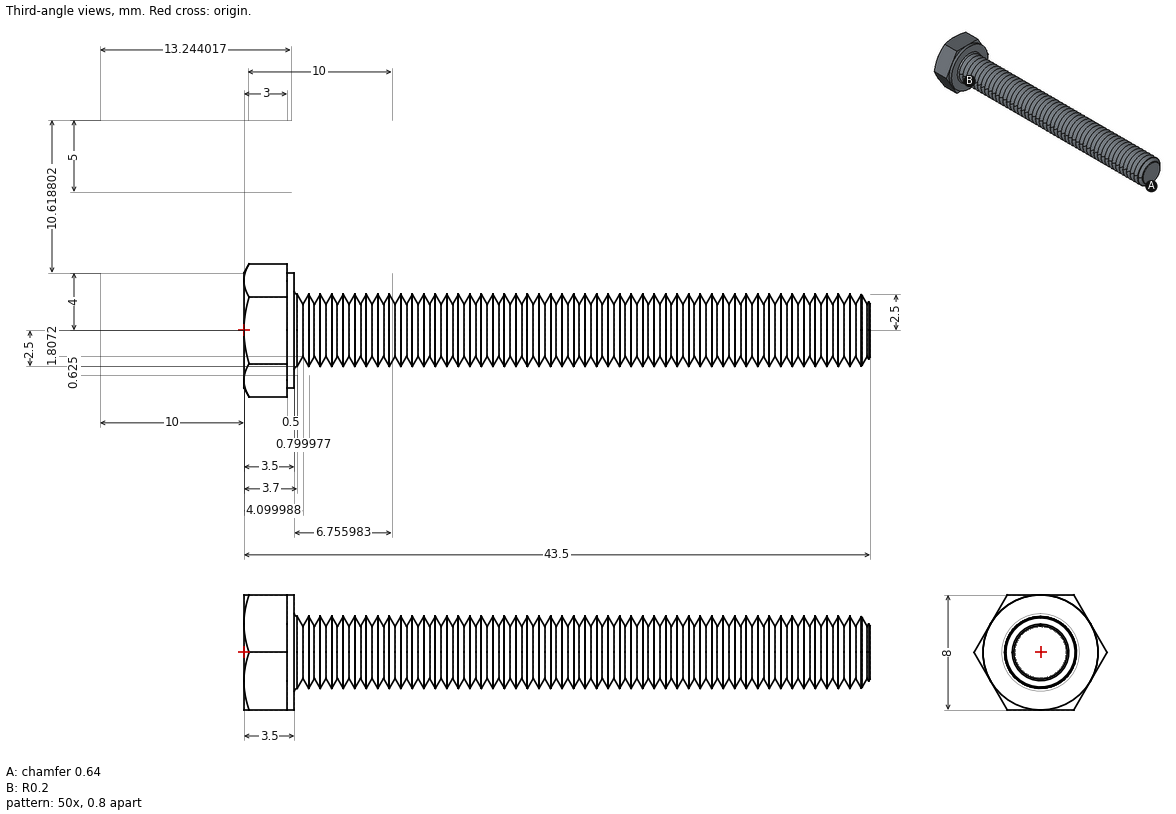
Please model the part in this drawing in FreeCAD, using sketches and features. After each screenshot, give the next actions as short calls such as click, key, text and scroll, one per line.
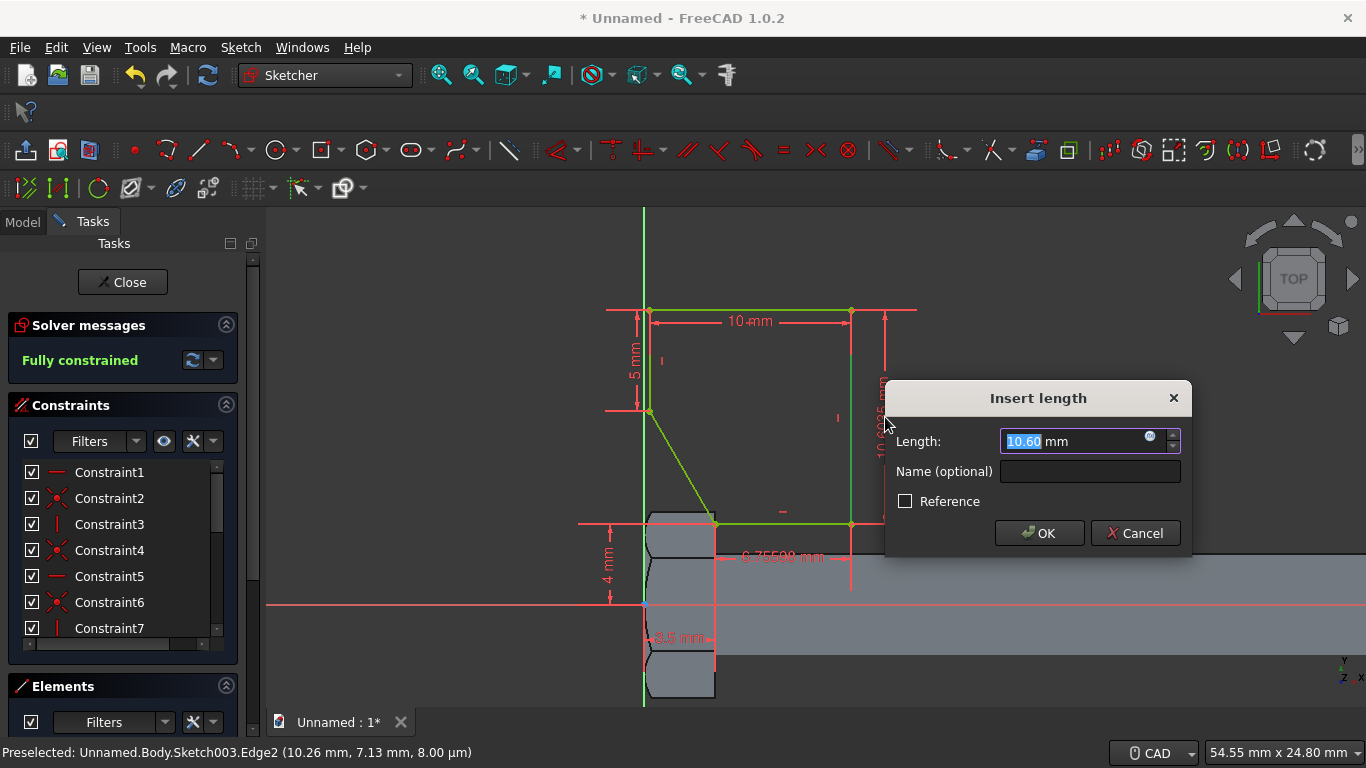
text(10.618802)
key(Return)
key(Escape)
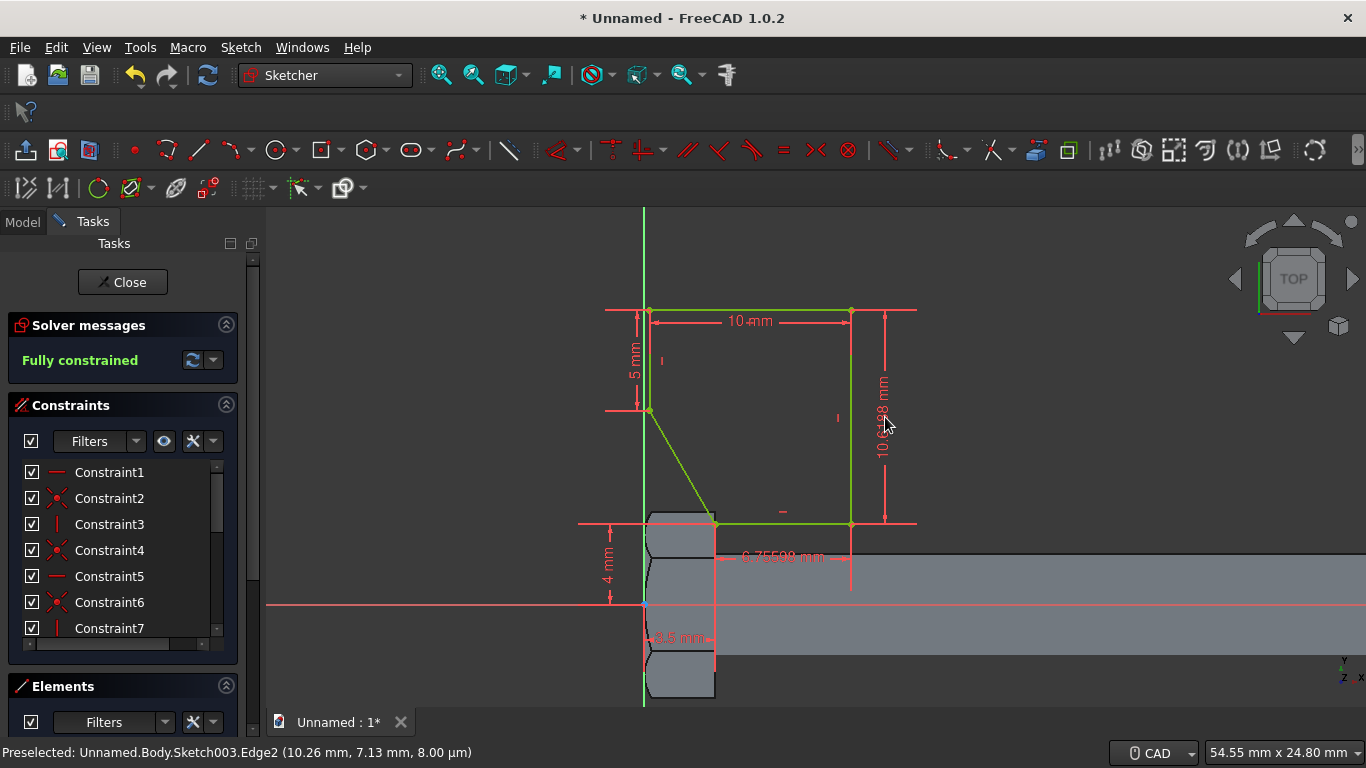
click(123, 282)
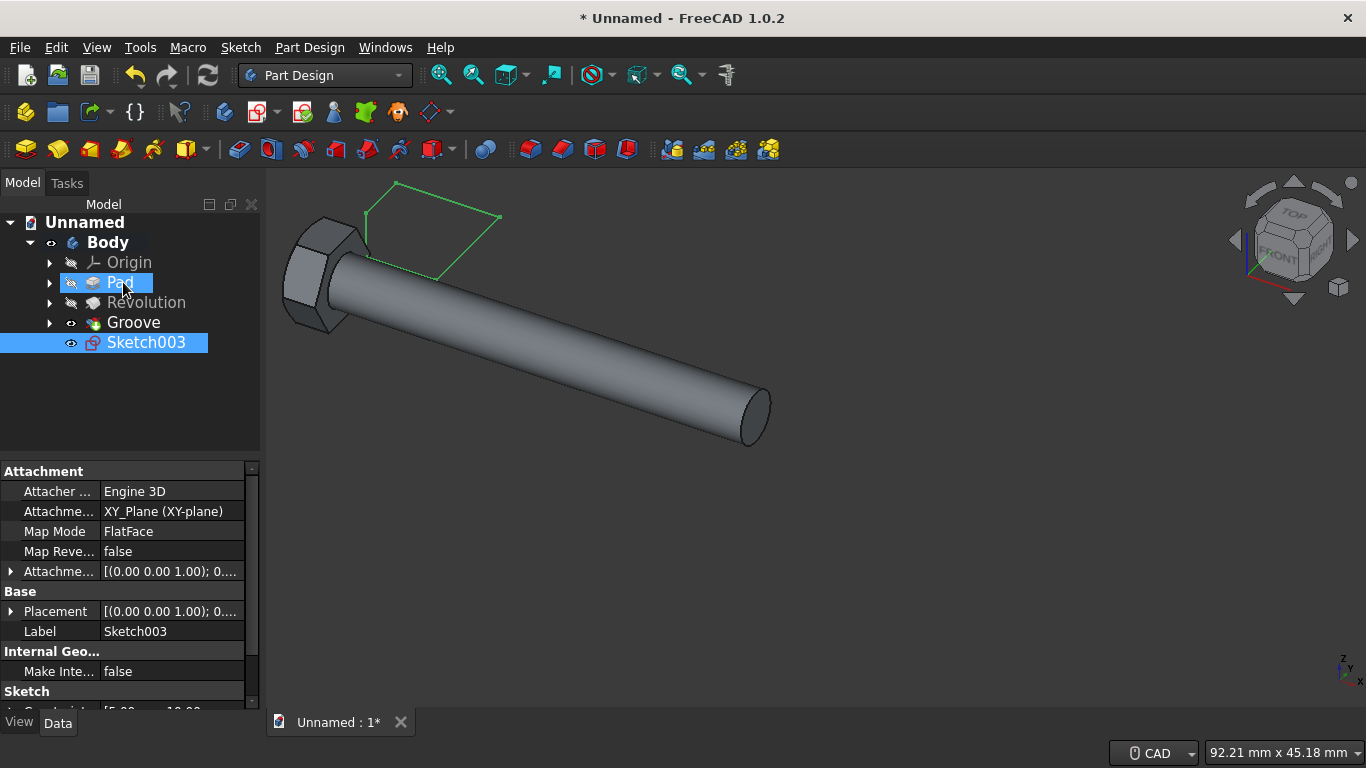
click(304, 150)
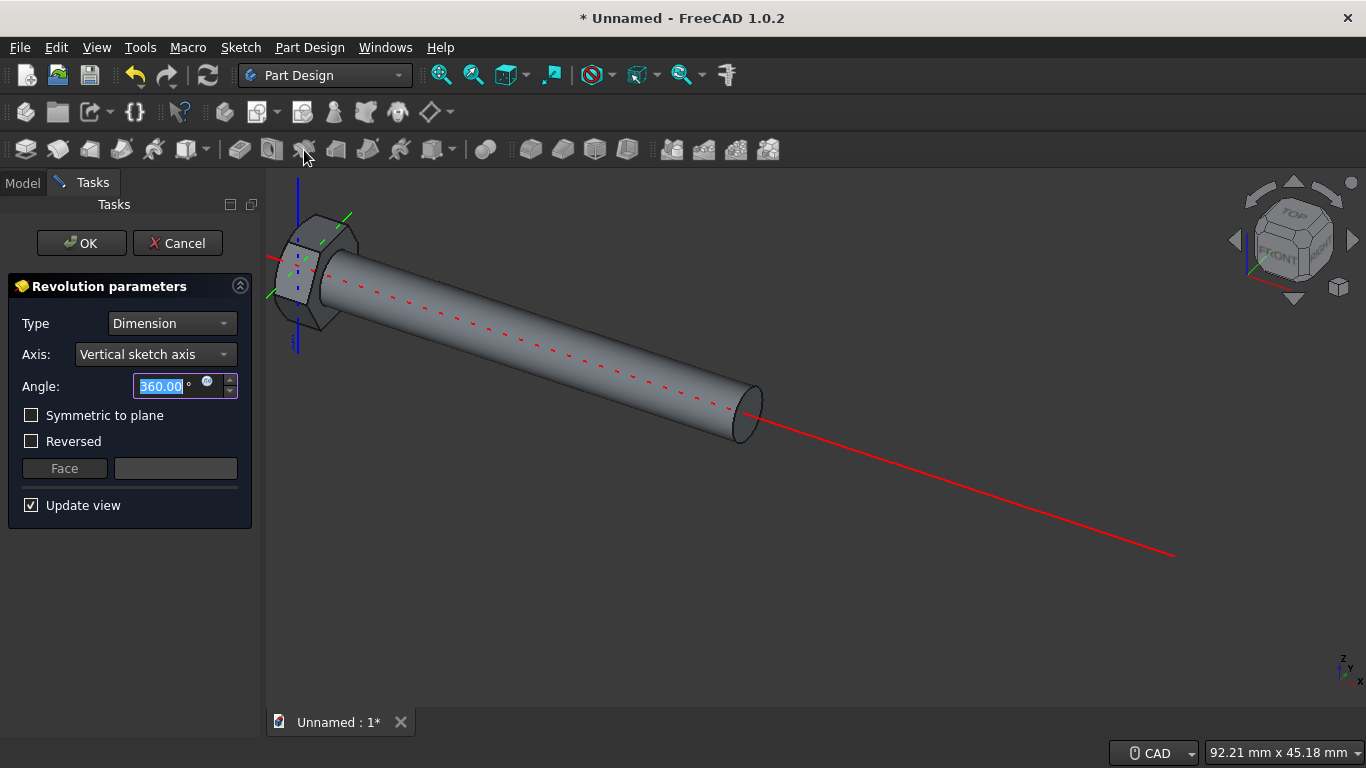
click(156, 354)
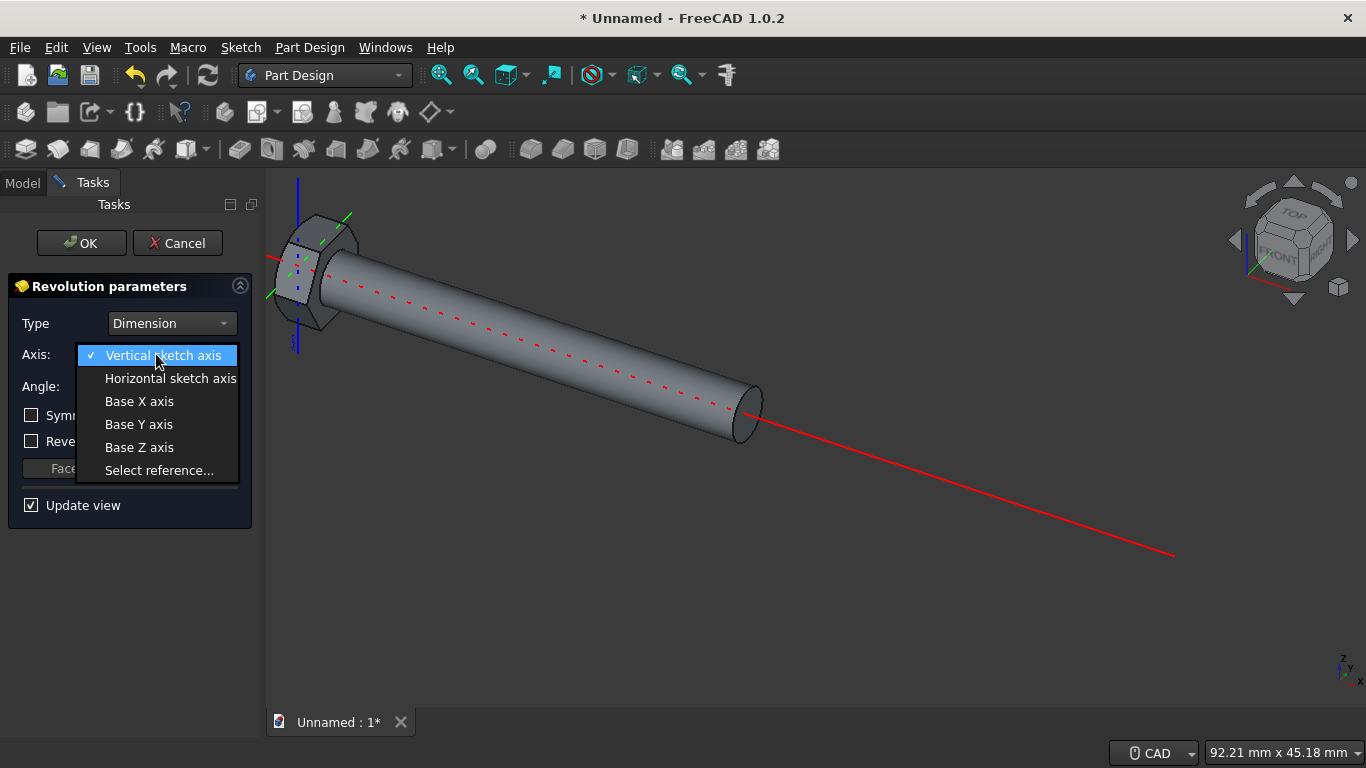
click(156, 378)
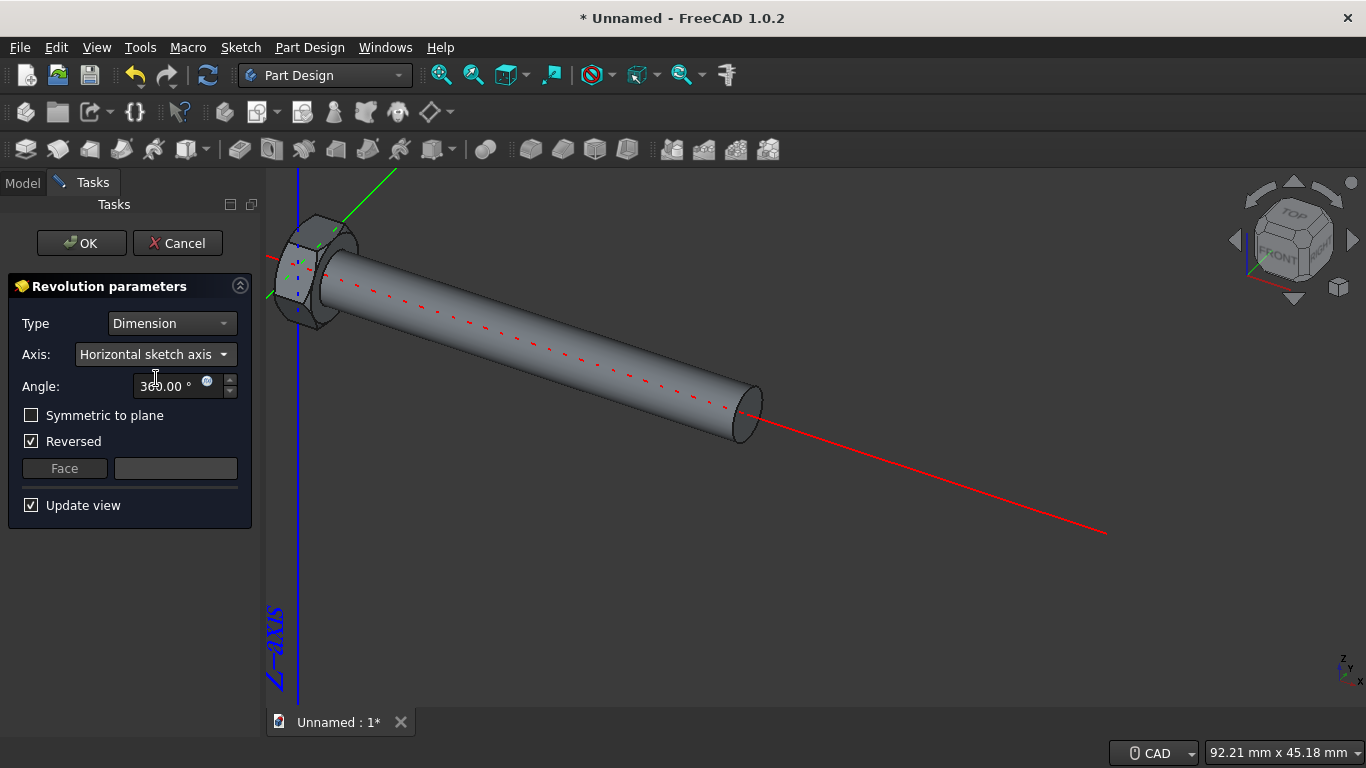
click(82, 243)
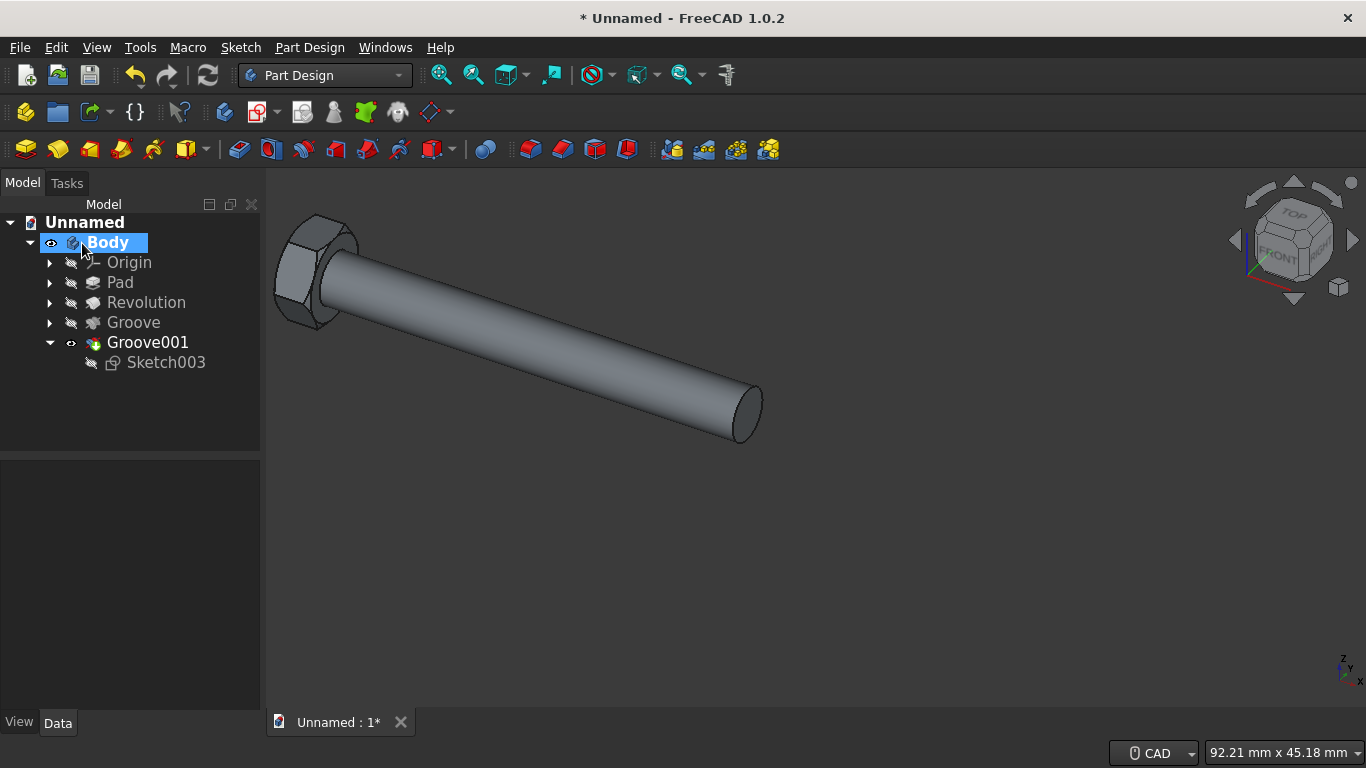
click(258, 112)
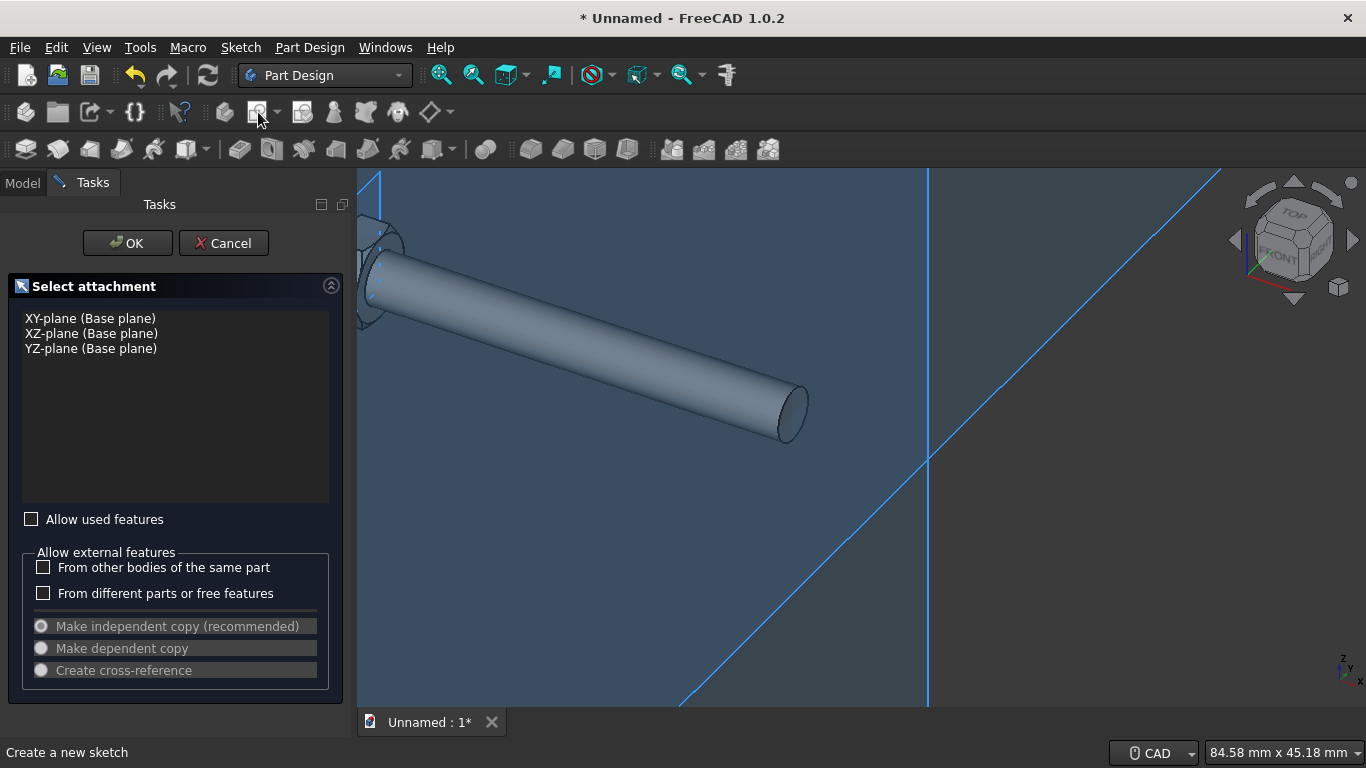
click(82, 318)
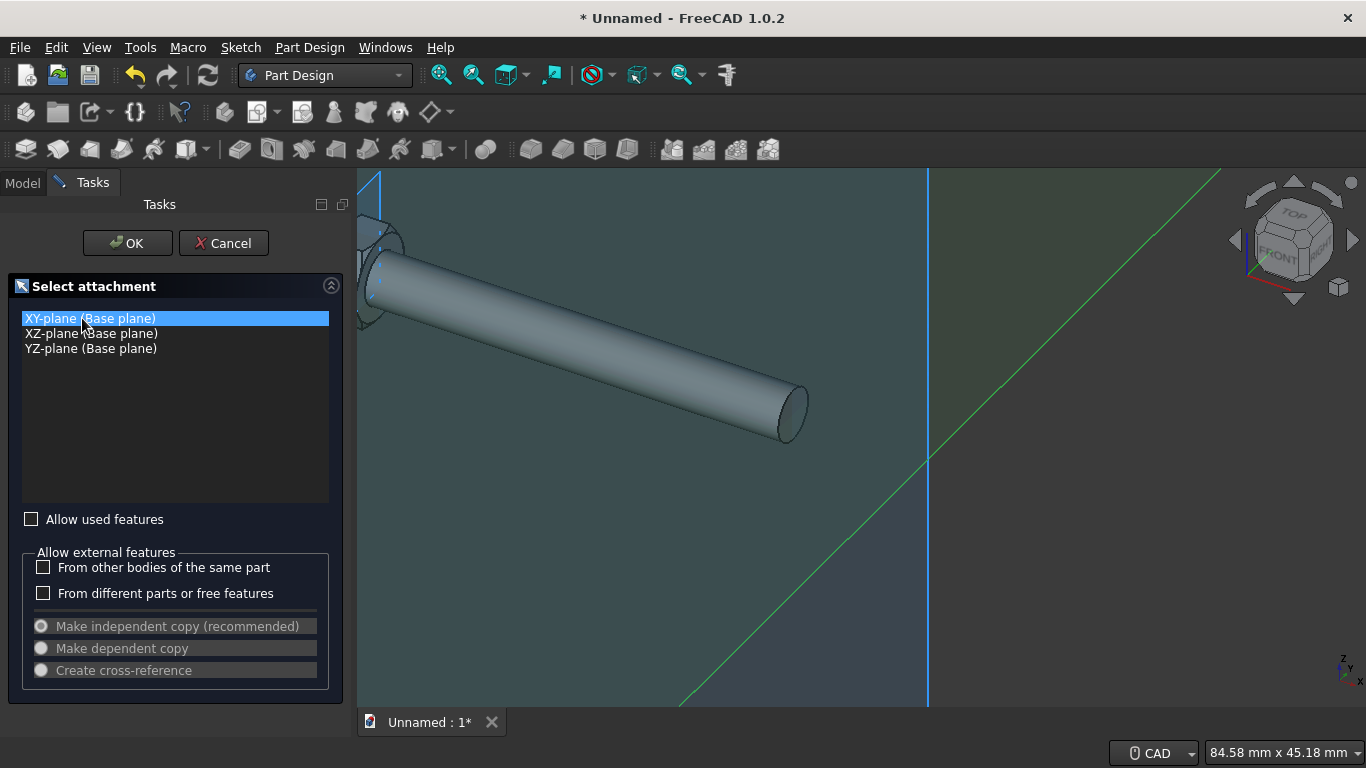
click(128, 243)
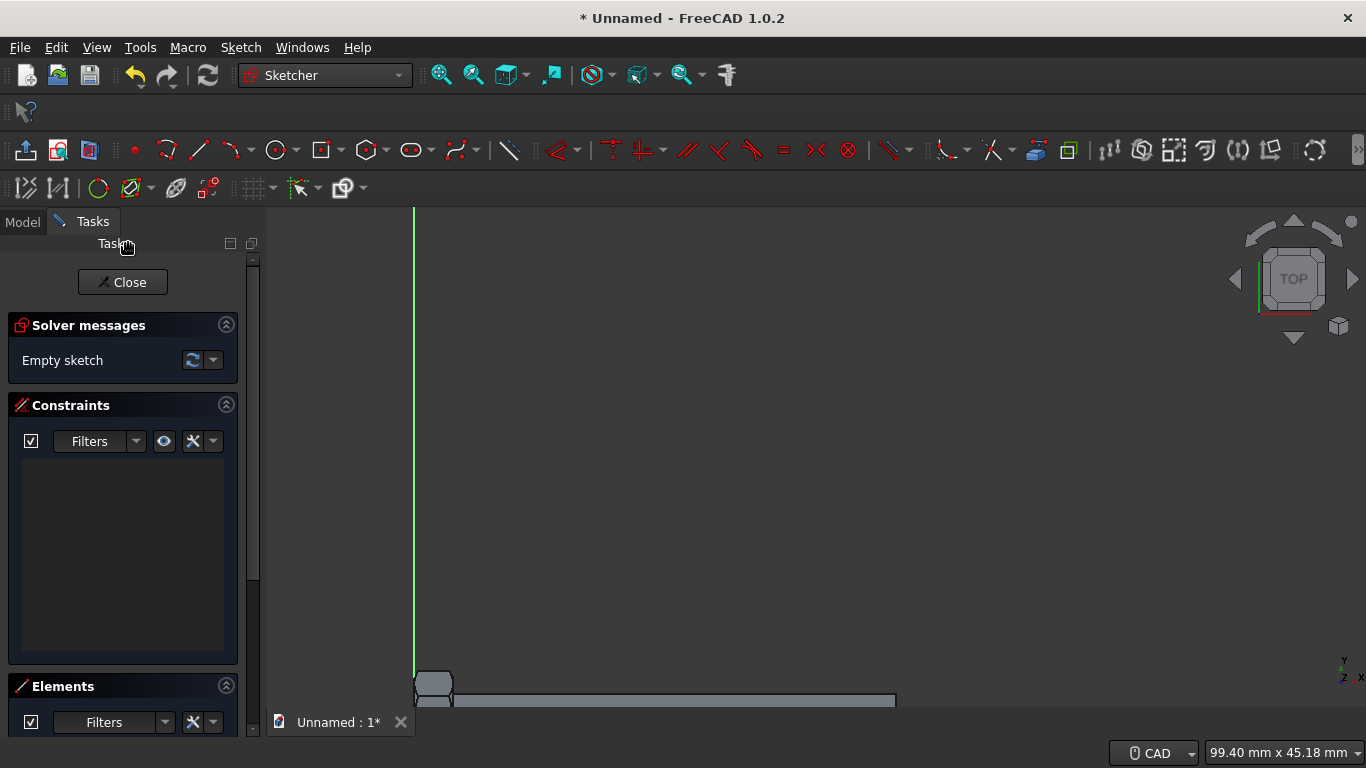
click(90, 150)